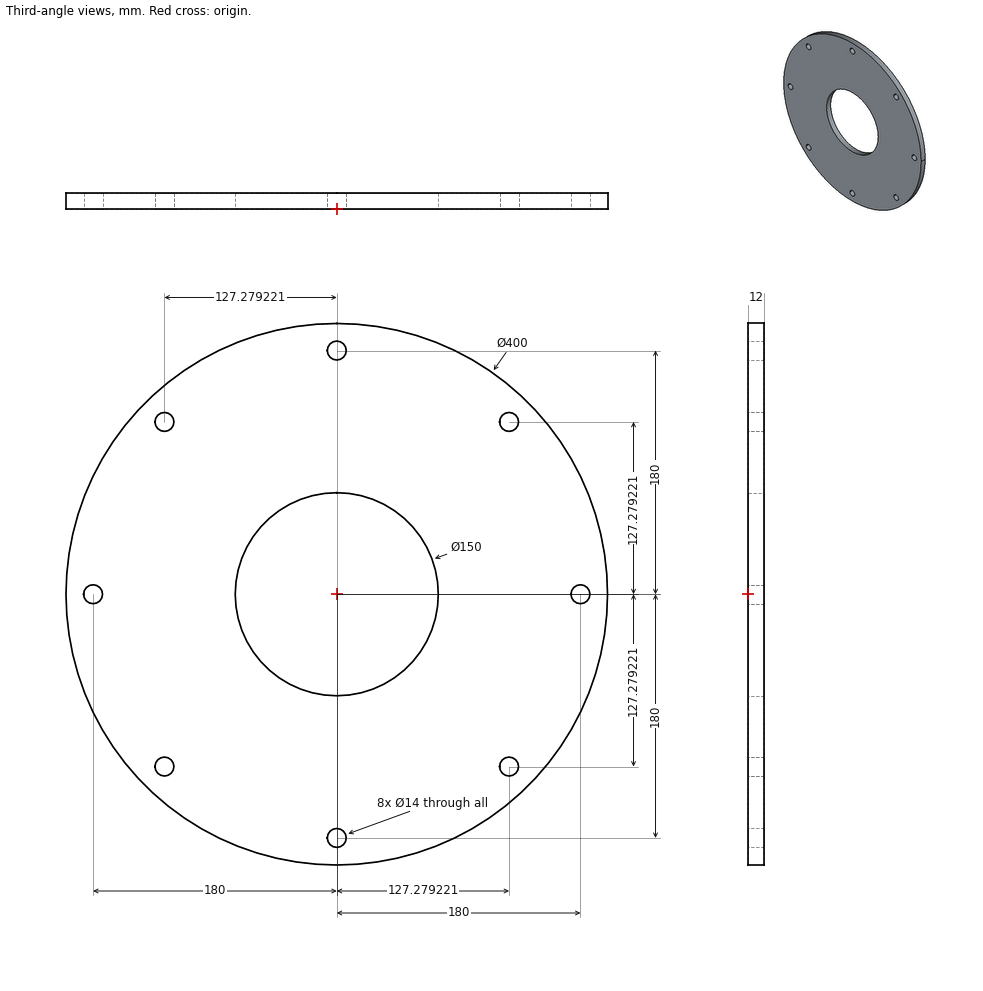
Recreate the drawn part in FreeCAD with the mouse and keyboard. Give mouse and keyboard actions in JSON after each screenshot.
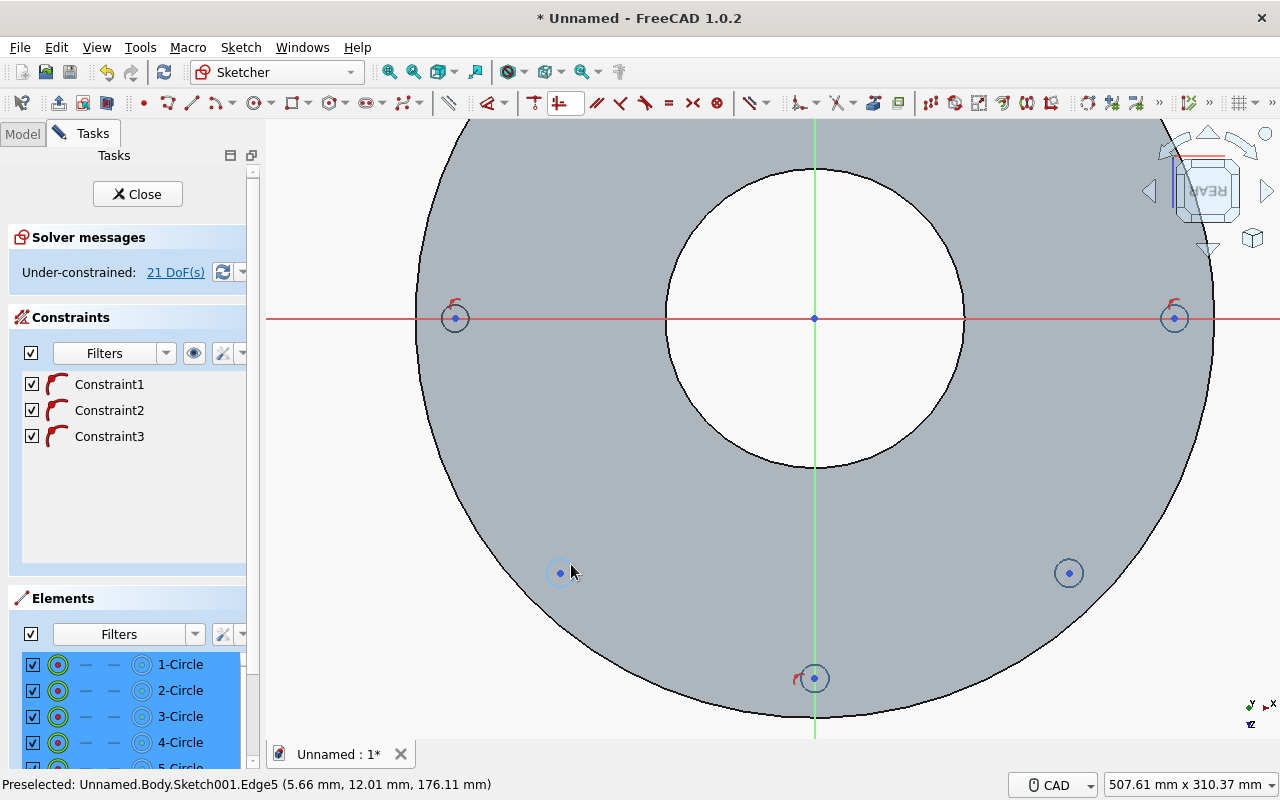
{"action": "left_click", "coordinate": [571, 563]}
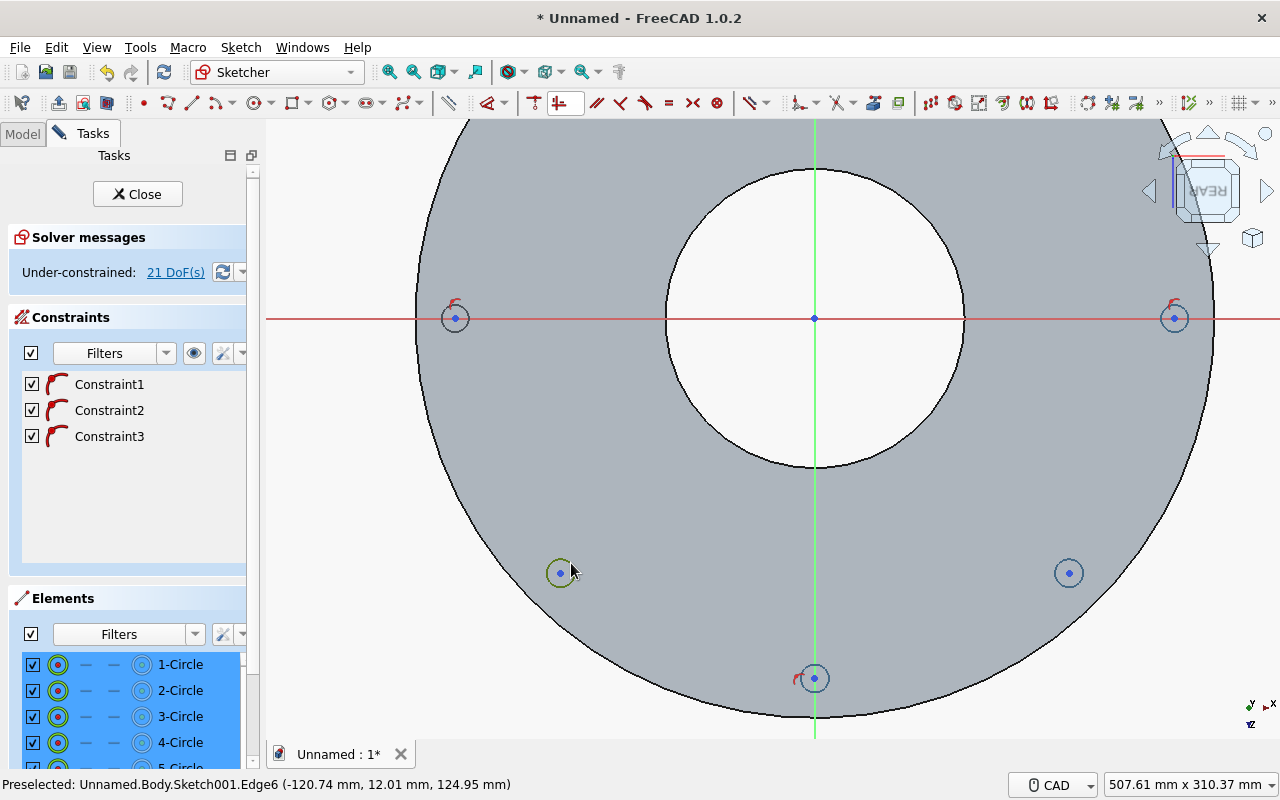
{"action": "scroll", "coordinate": [465, 309], "scroll_direction": "up", "scroll_amount": 2}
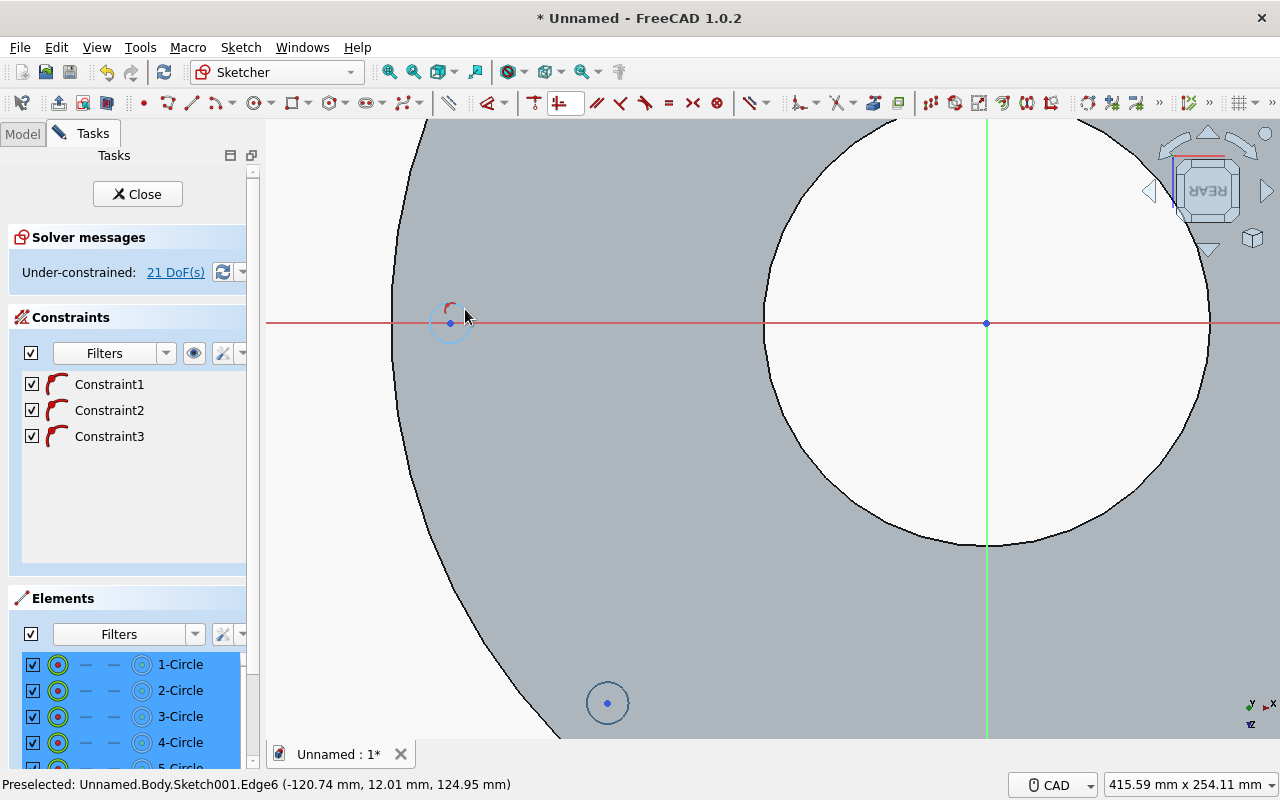
{"action": "left_click", "coordinate": [464, 309]}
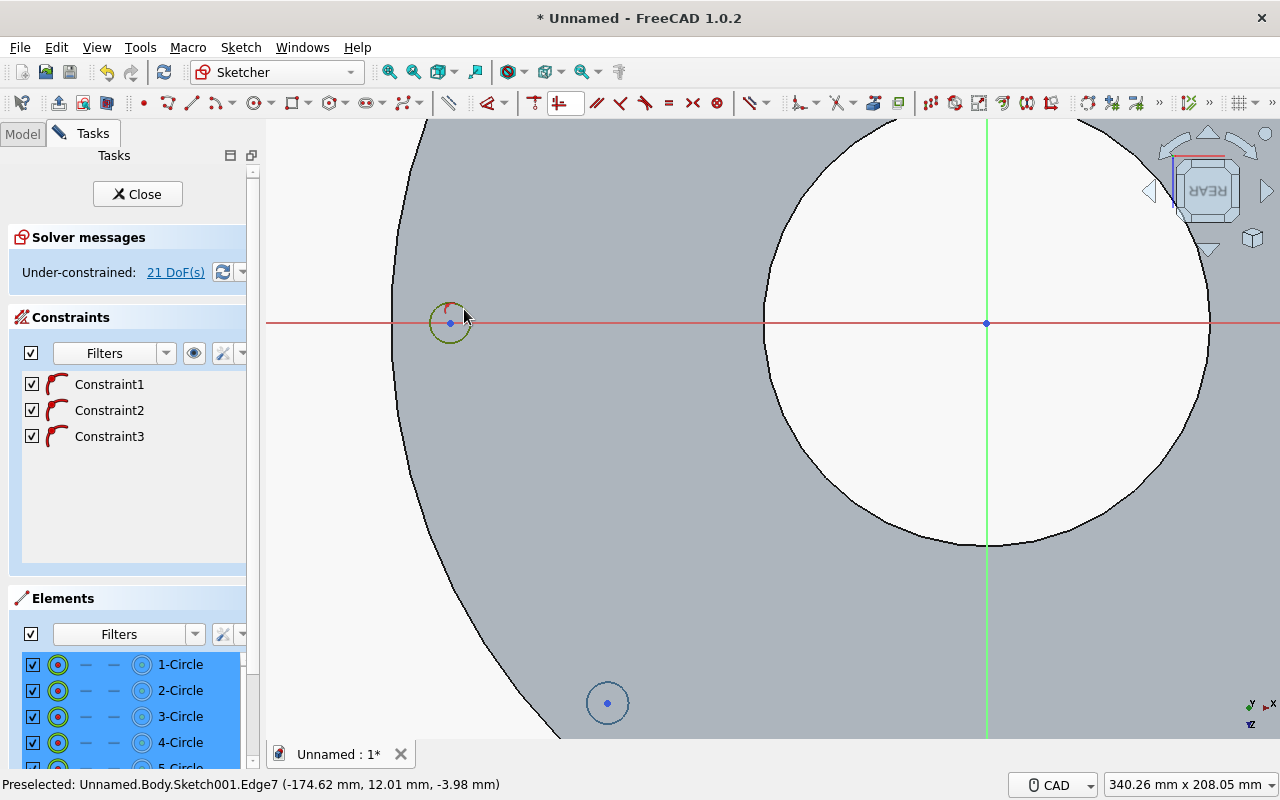
{"action": "scroll", "coordinate": [540, 491], "scroll_direction": "down", "scroll_amount": 5}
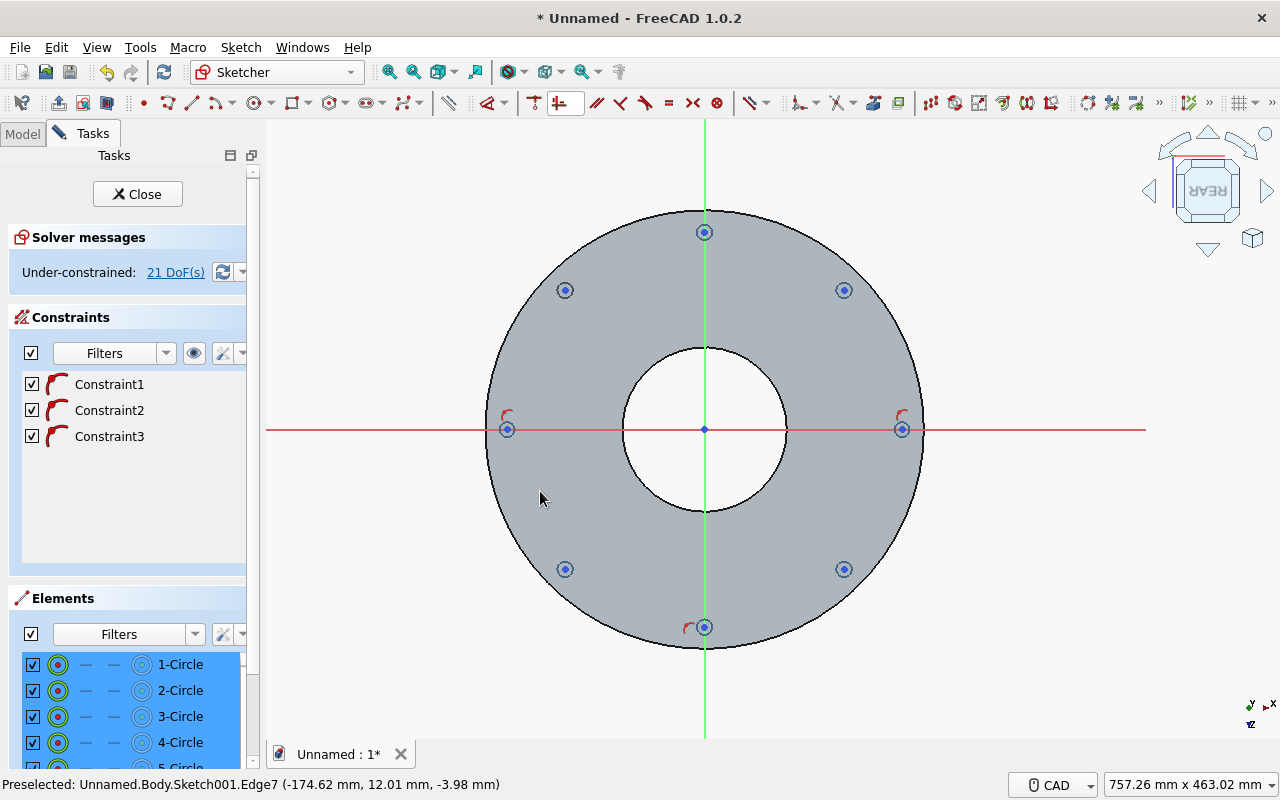
{"action": "scroll", "coordinate": [570, 285], "scroll_direction": "up", "scroll_amount": 3}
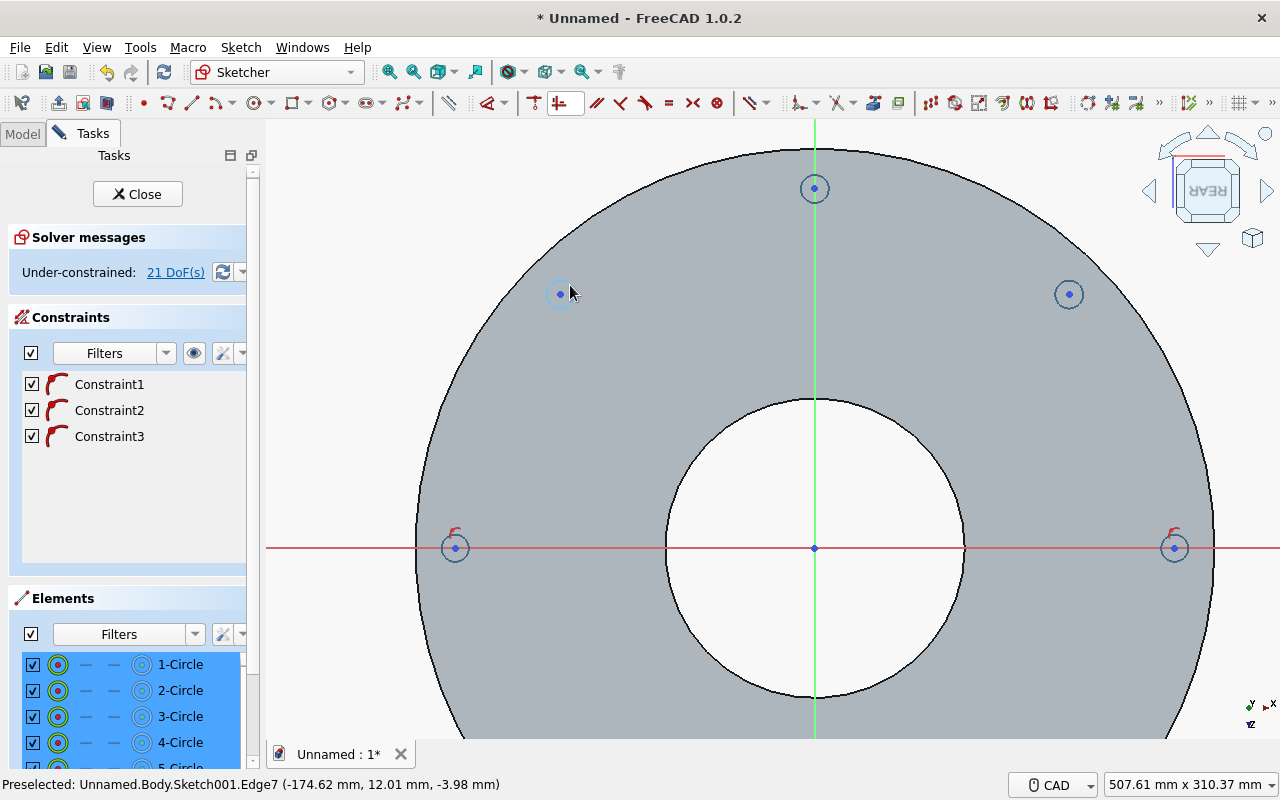
{"action": "left_click", "coordinate": [571, 285]}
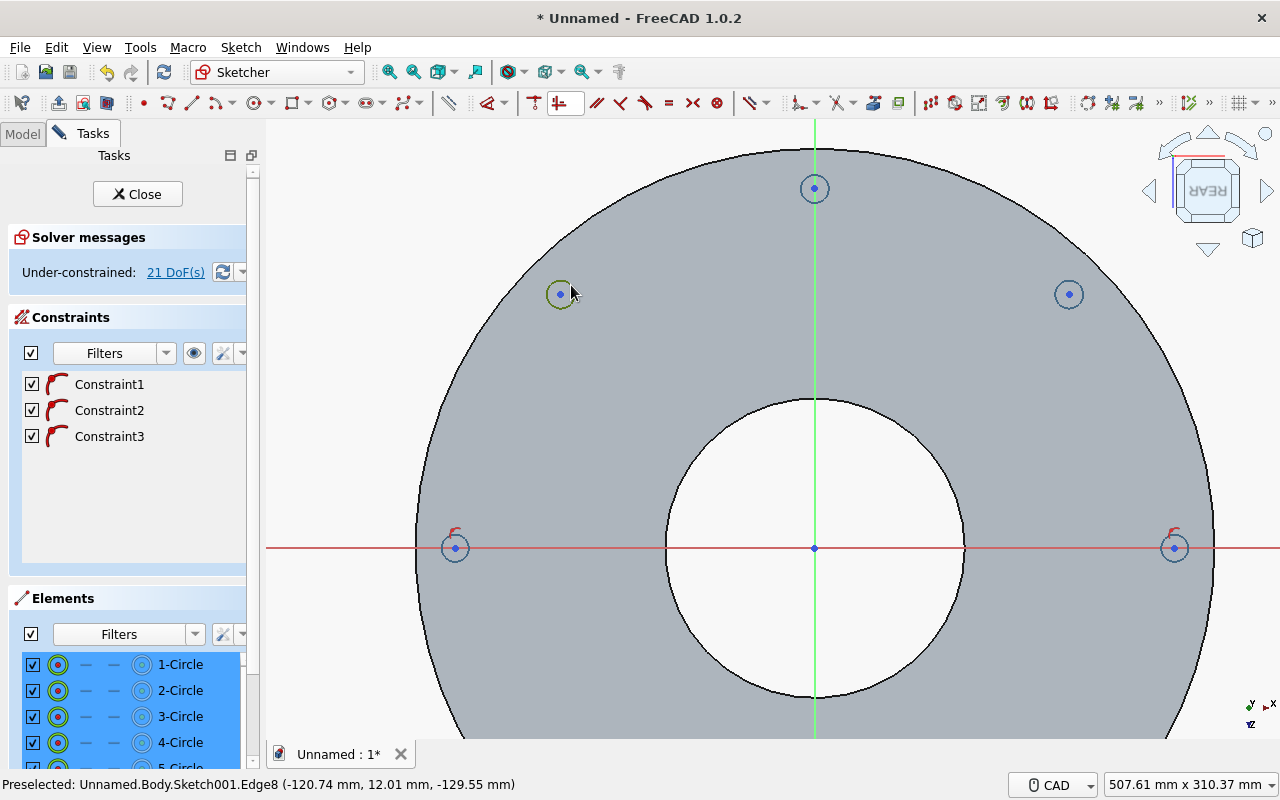
{"action": "left_click", "coordinate": [670, 104]}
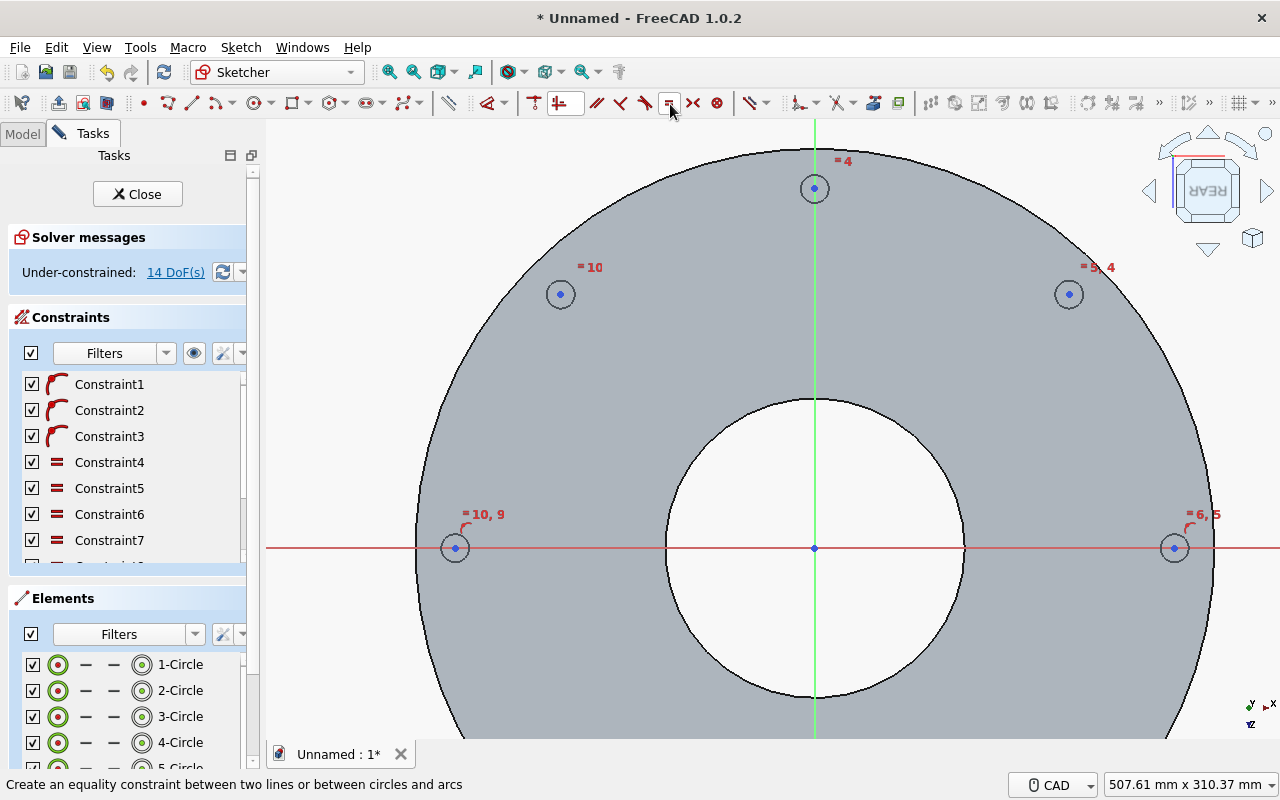
{"action": "left_click", "coordinate": [815, 189]}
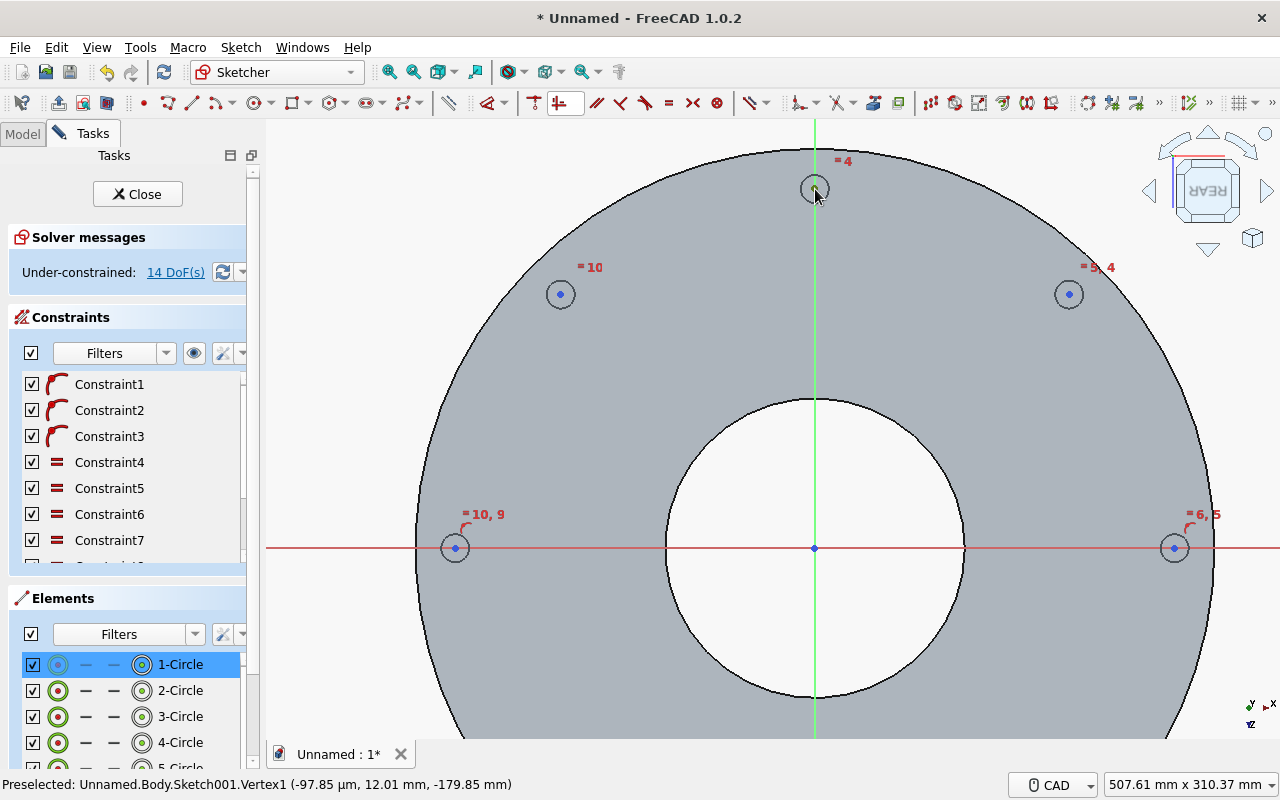
{"action": "left_click", "coordinate": [815, 671]}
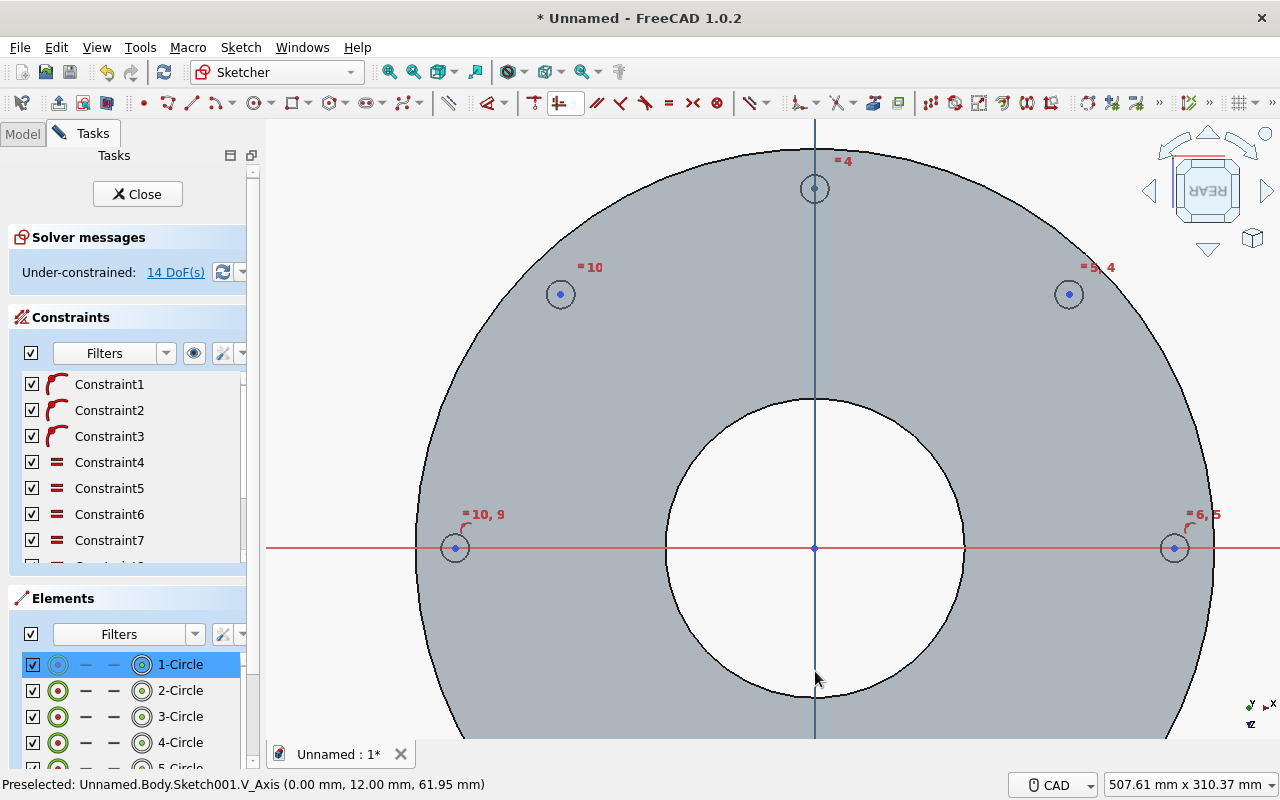
{"action": "left_click", "coordinate": [534, 104]}